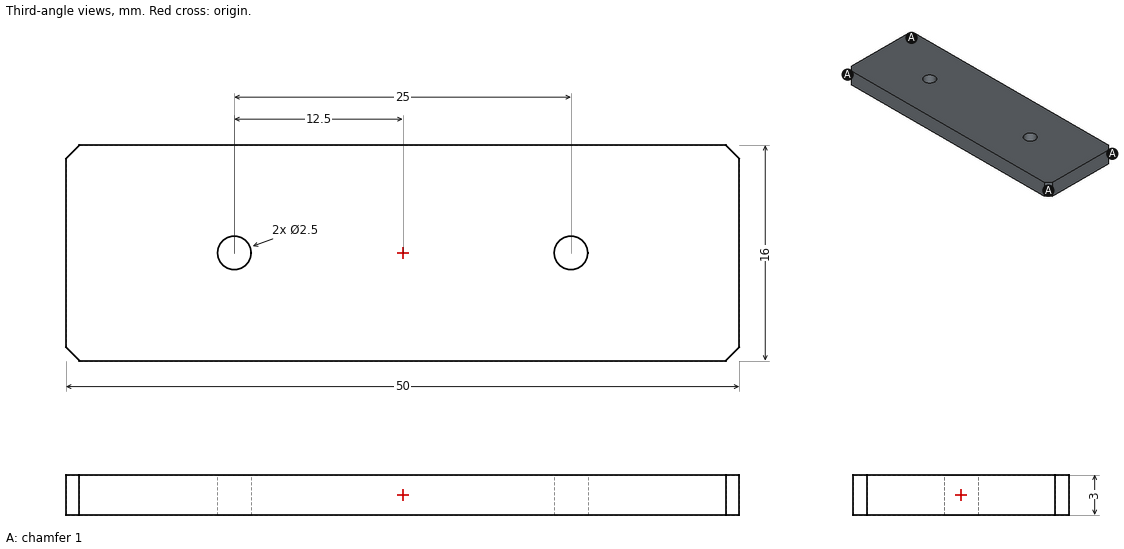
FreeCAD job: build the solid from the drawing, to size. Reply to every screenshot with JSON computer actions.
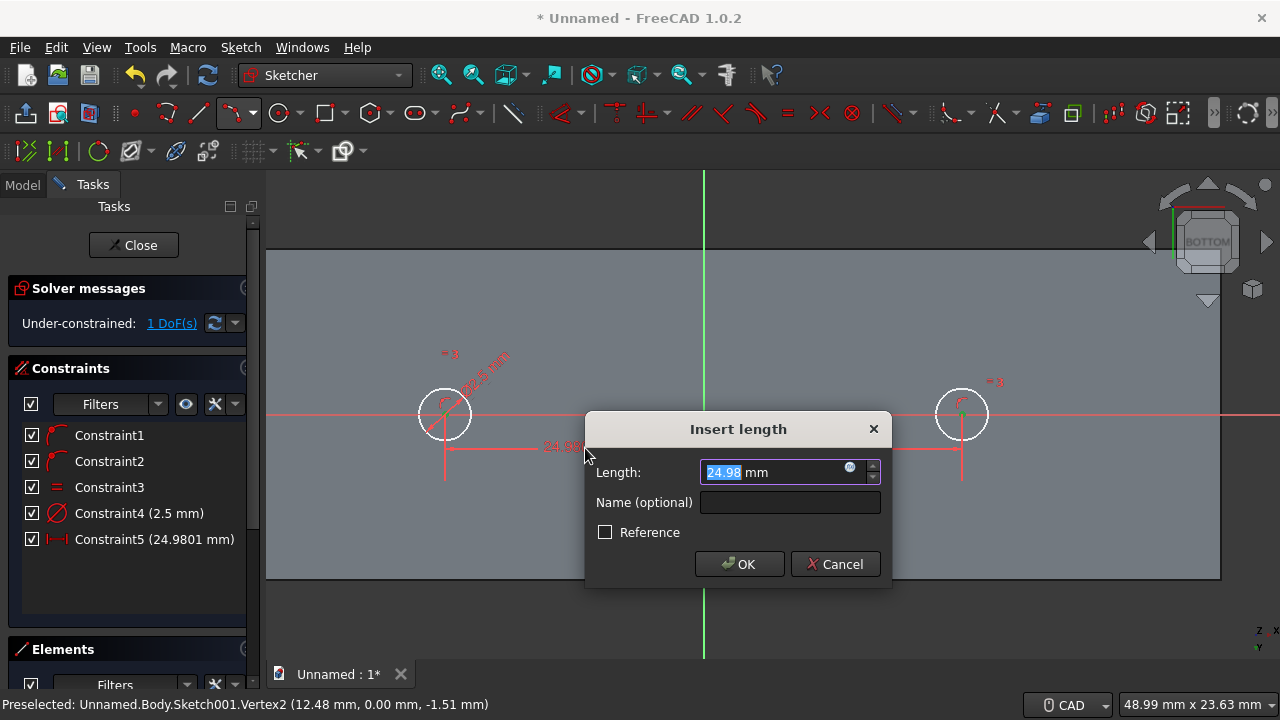
{"action": "type", "text": "25"}
{"action": "key", "text": "Return"}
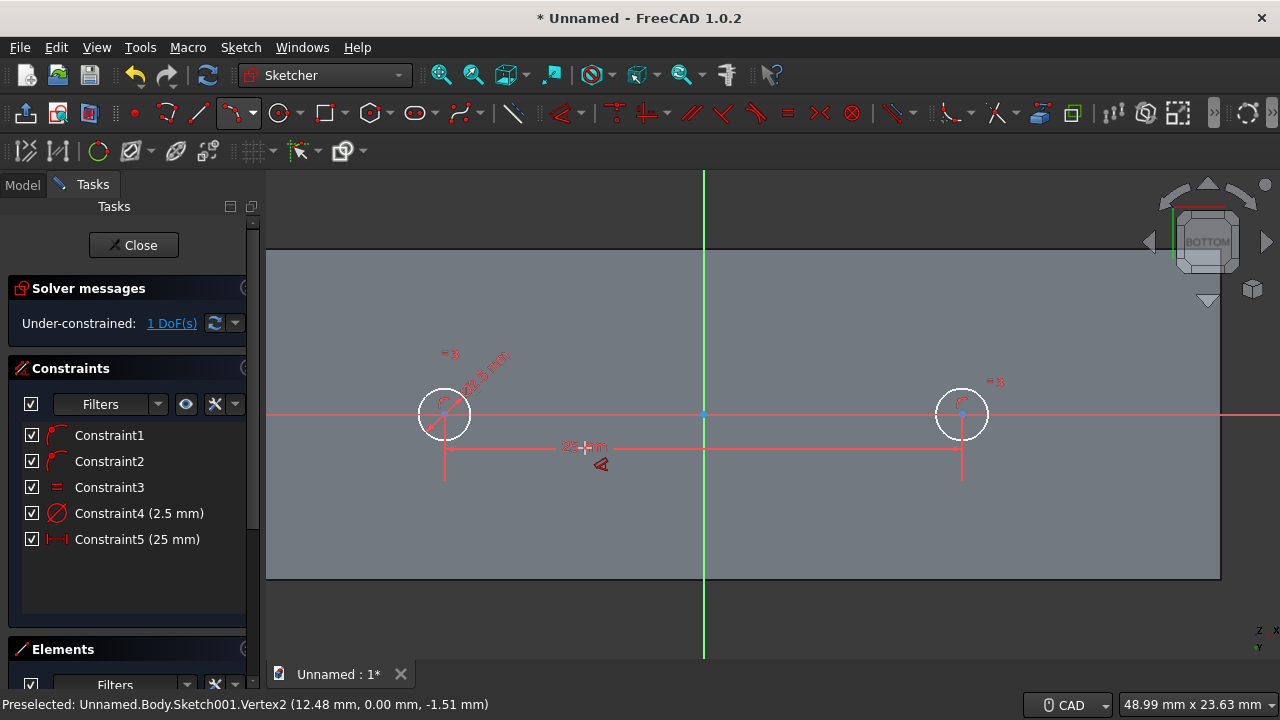
{"action": "left_click", "coordinate": [445, 414]}
{"action": "left_click", "coordinate": [515, 448]}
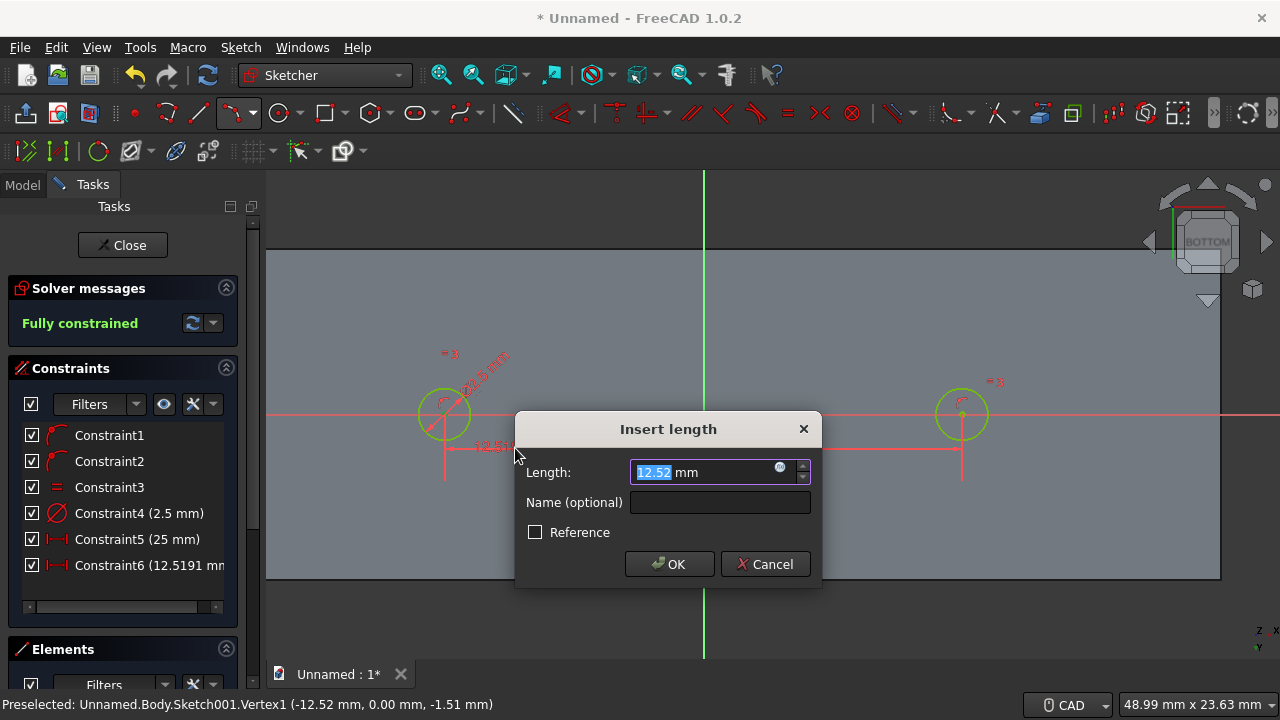
{"action": "type", "text": "12.5"}
{"action": "key", "text": "Return"}
{"action": "key", "text": "Escape"}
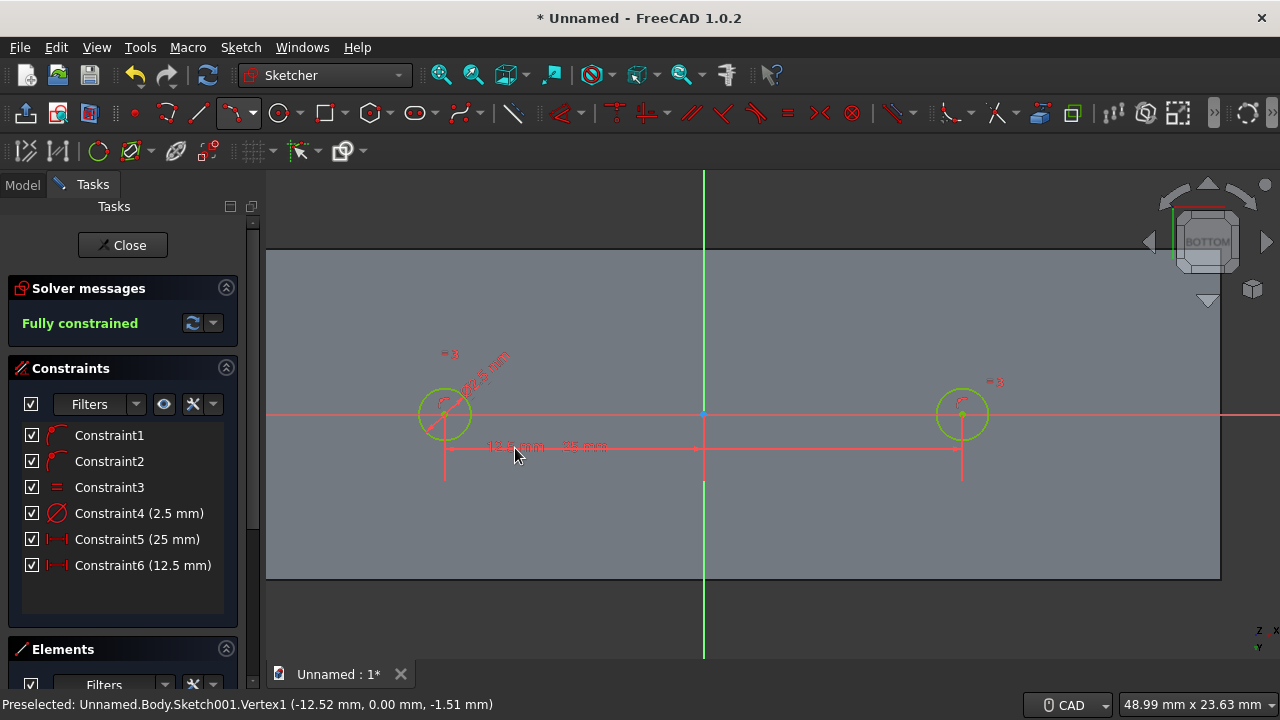
{"action": "left_click", "coordinate": [123, 245]}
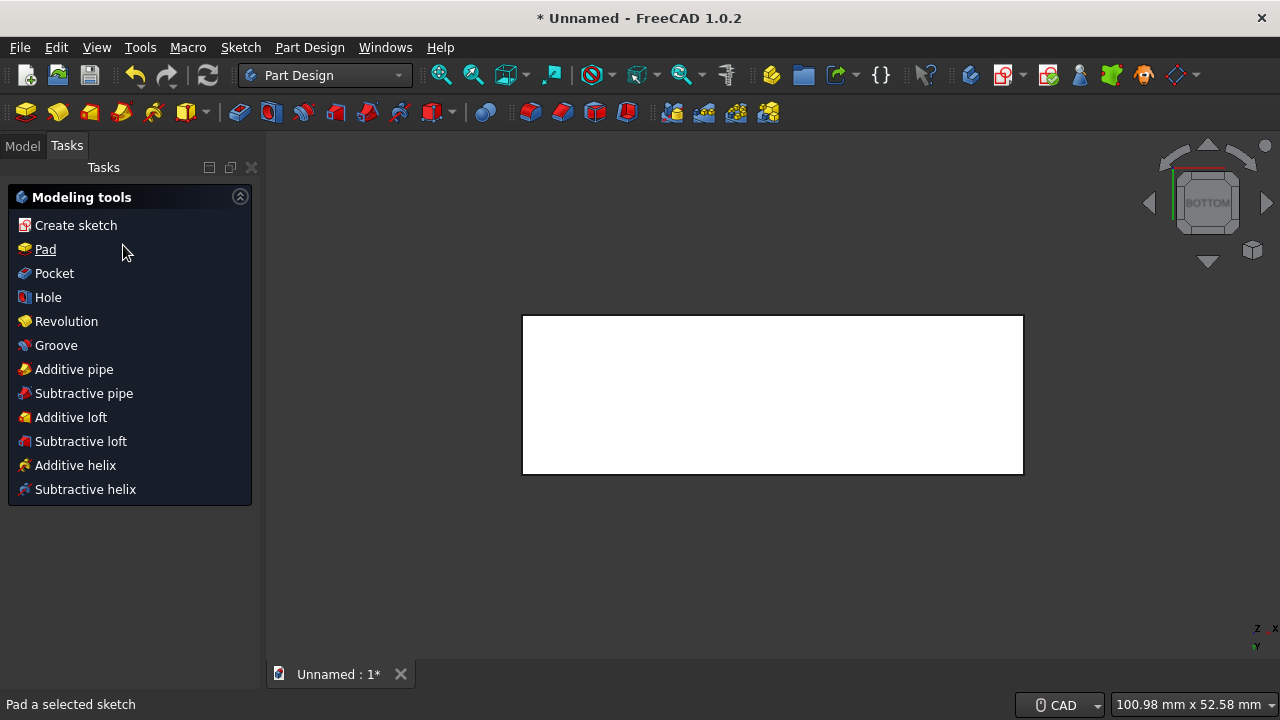
{"action": "left_click", "coordinate": [240, 112]}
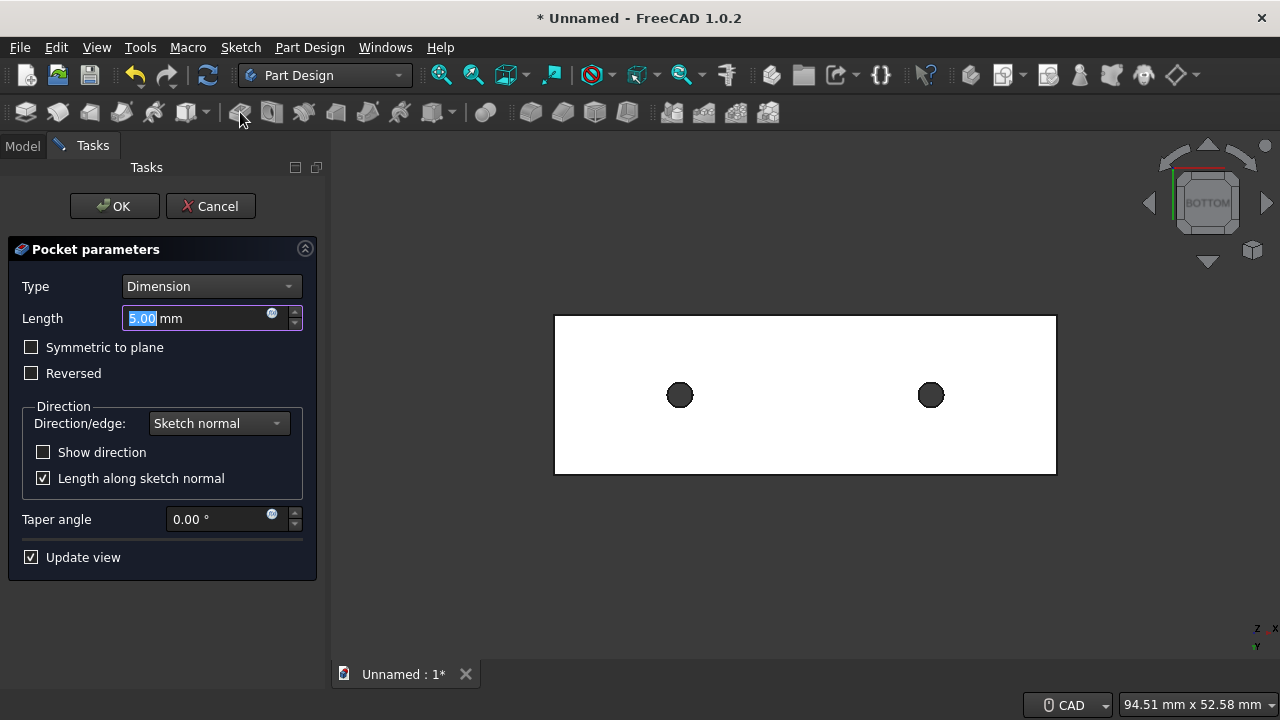
{"action": "left_click", "coordinate": [212, 286]}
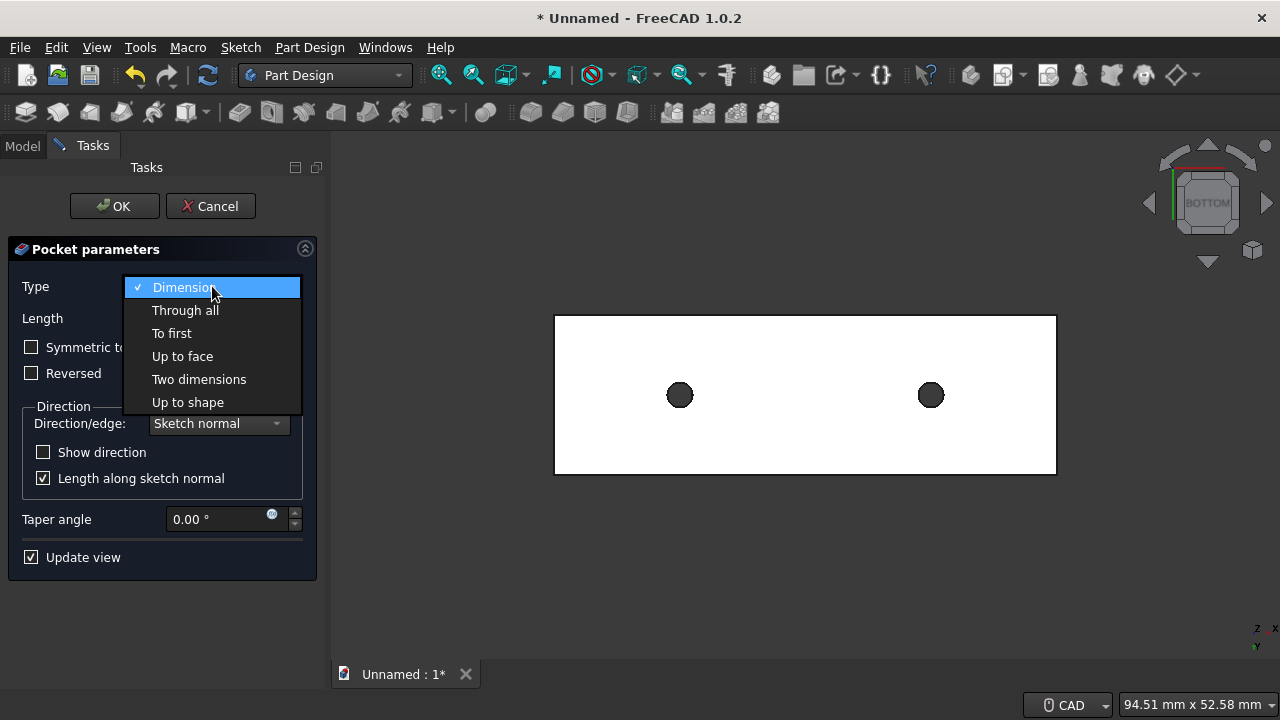
{"action": "left_click", "coordinate": [212, 310]}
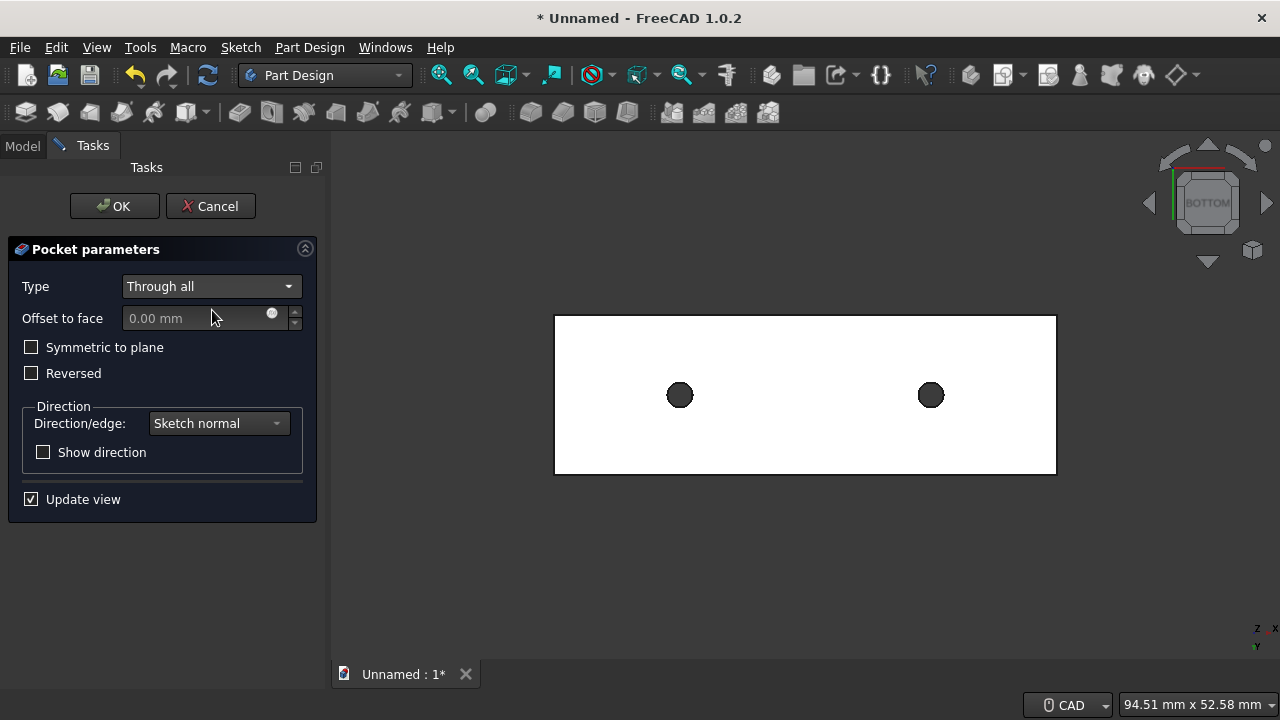
{"action": "left_click", "coordinate": [115, 206]}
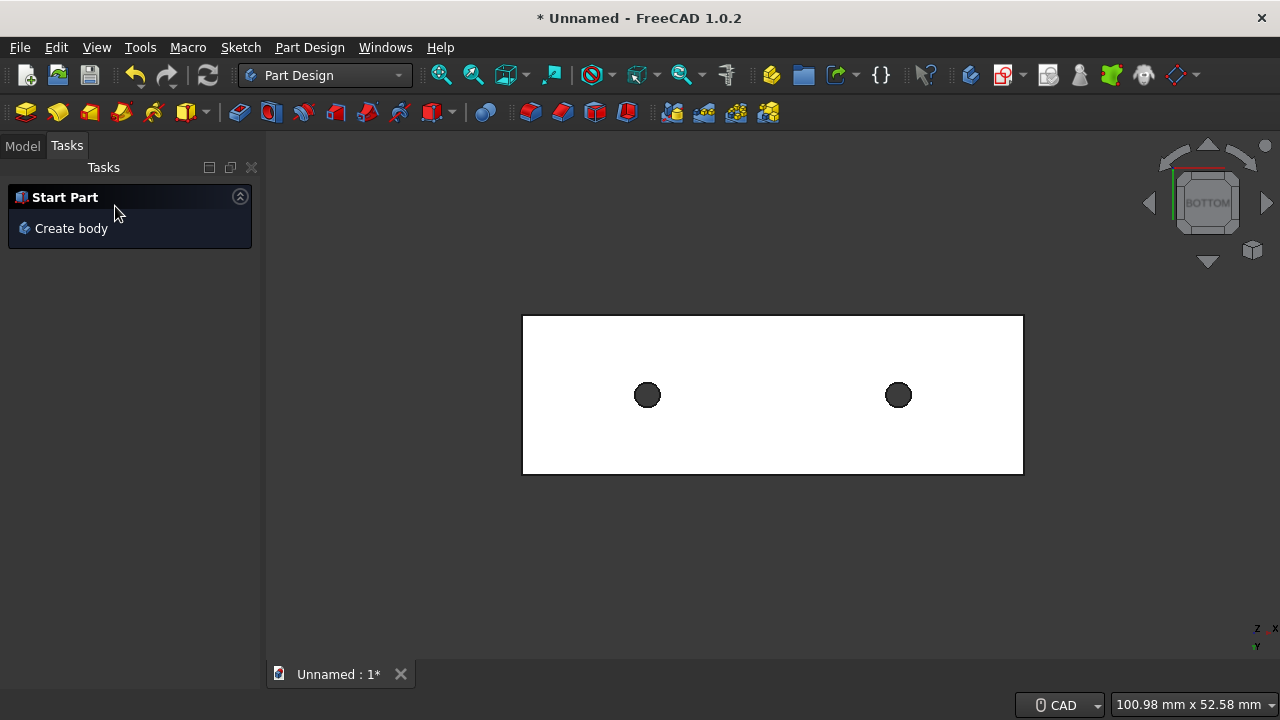
{"action": "key", "text": "0"}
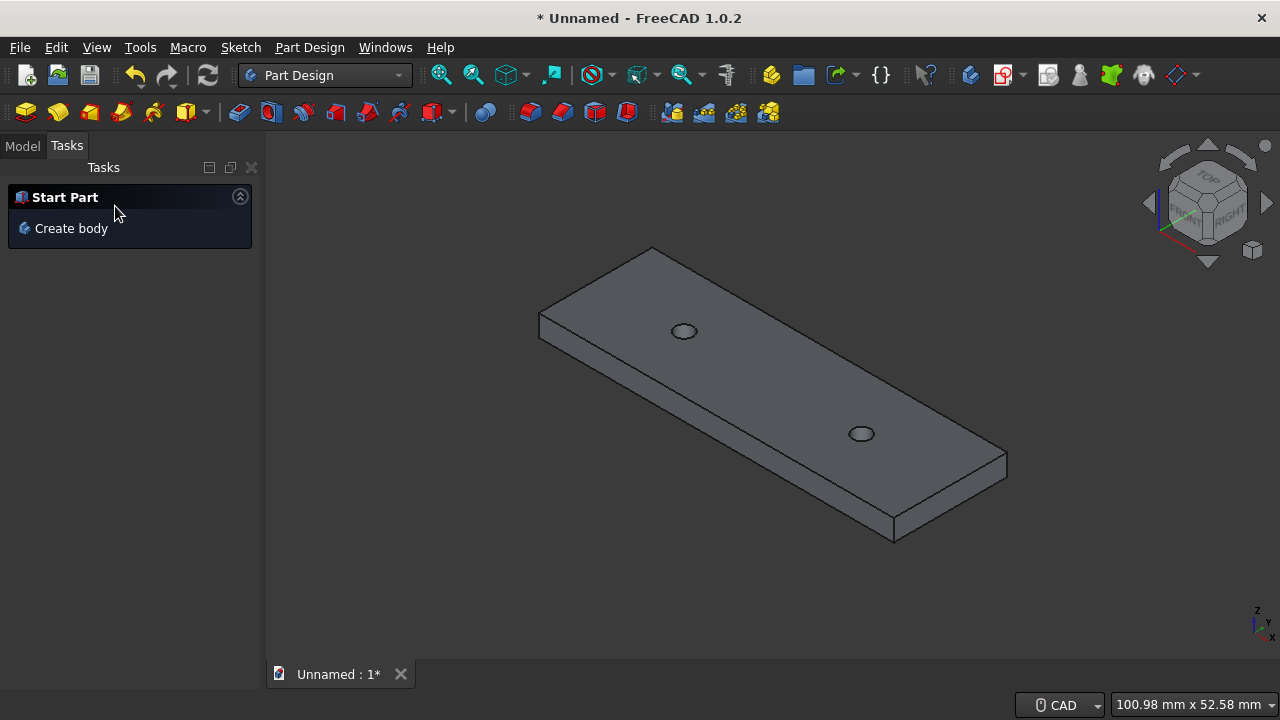
{"action": "left_click", "coordinate": [894, 529]}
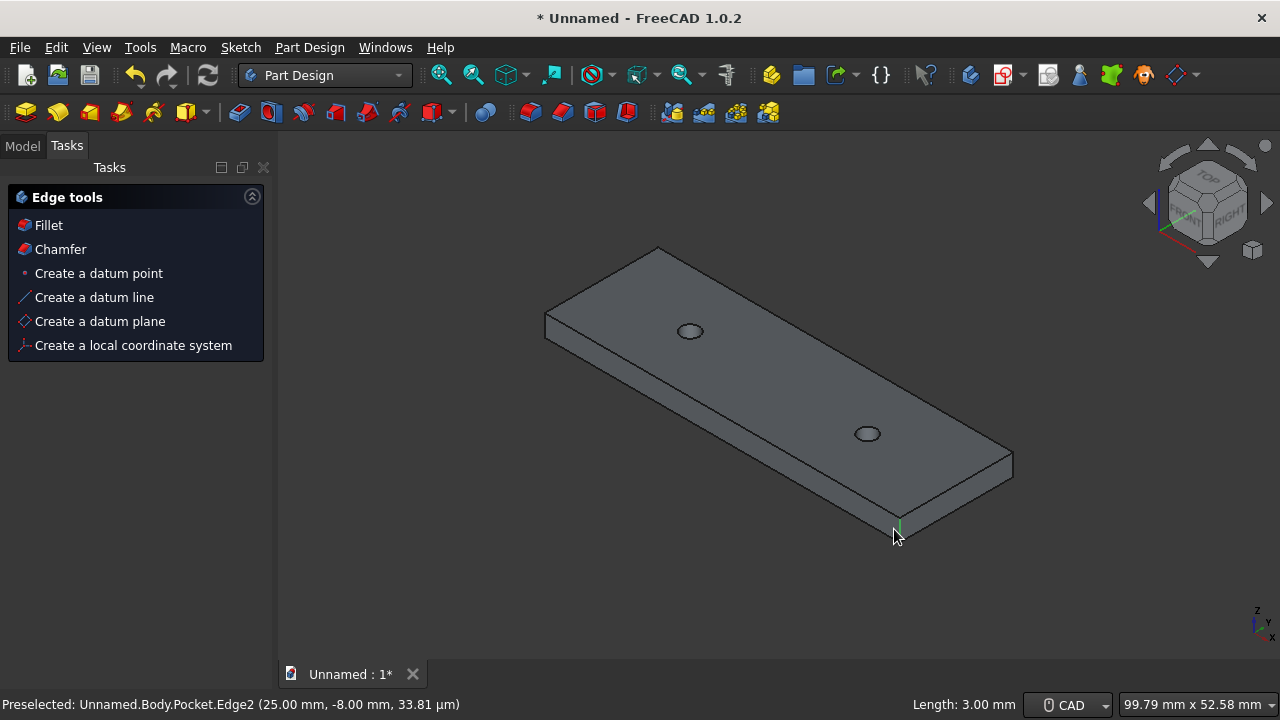
{"action": "key", "text": "2"}